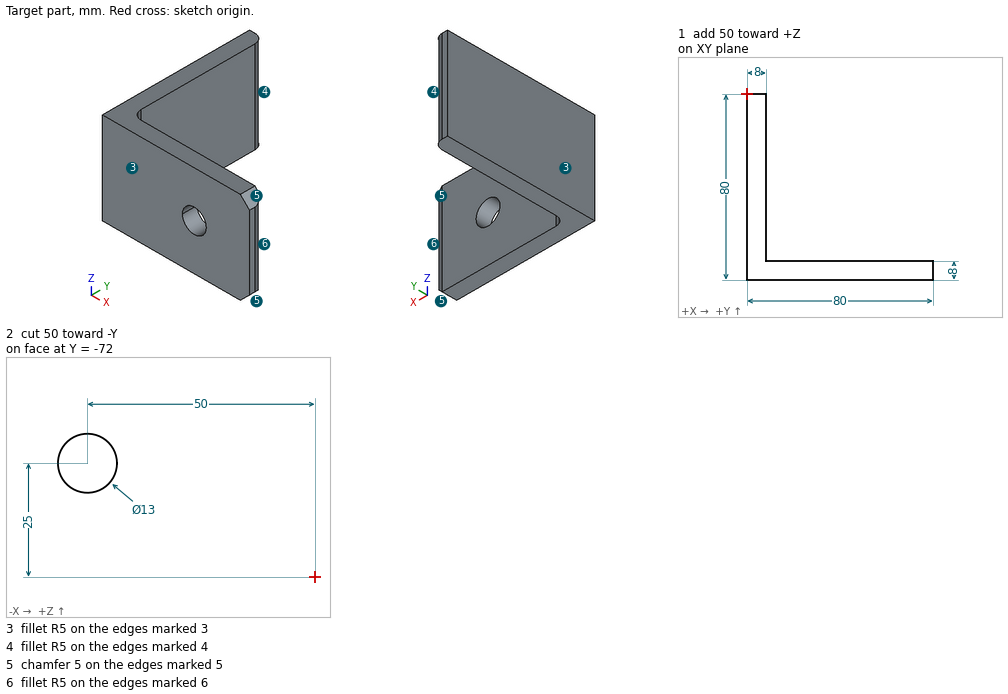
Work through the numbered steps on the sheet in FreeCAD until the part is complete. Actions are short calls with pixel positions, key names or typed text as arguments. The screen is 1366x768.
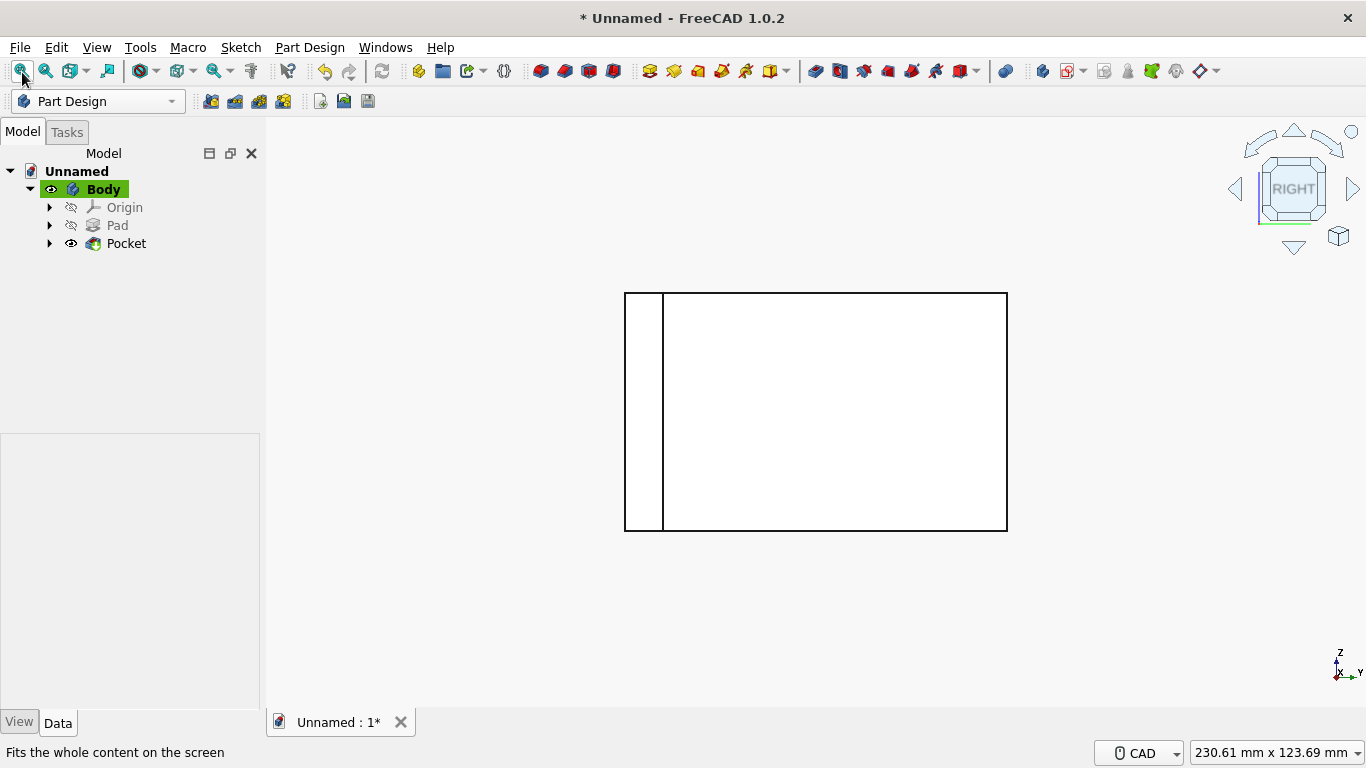
key(5)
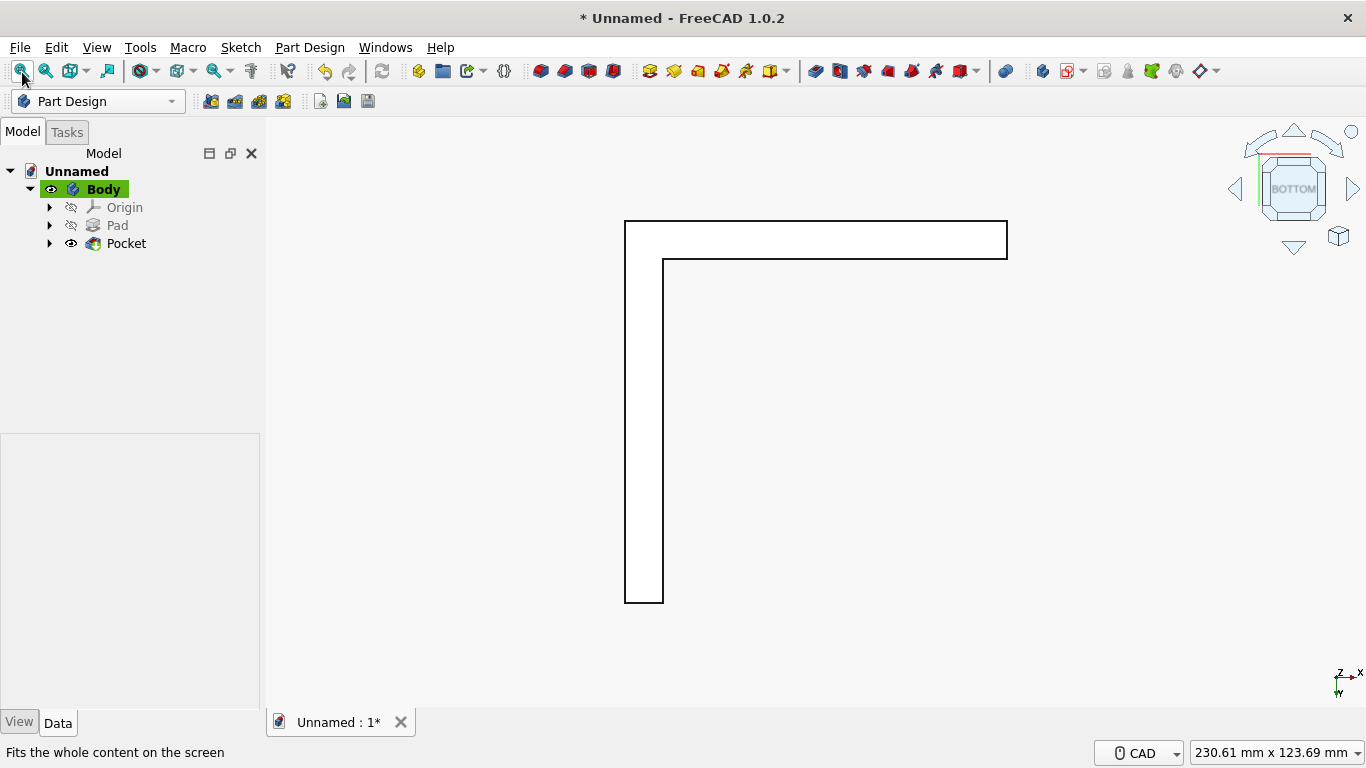
key(4)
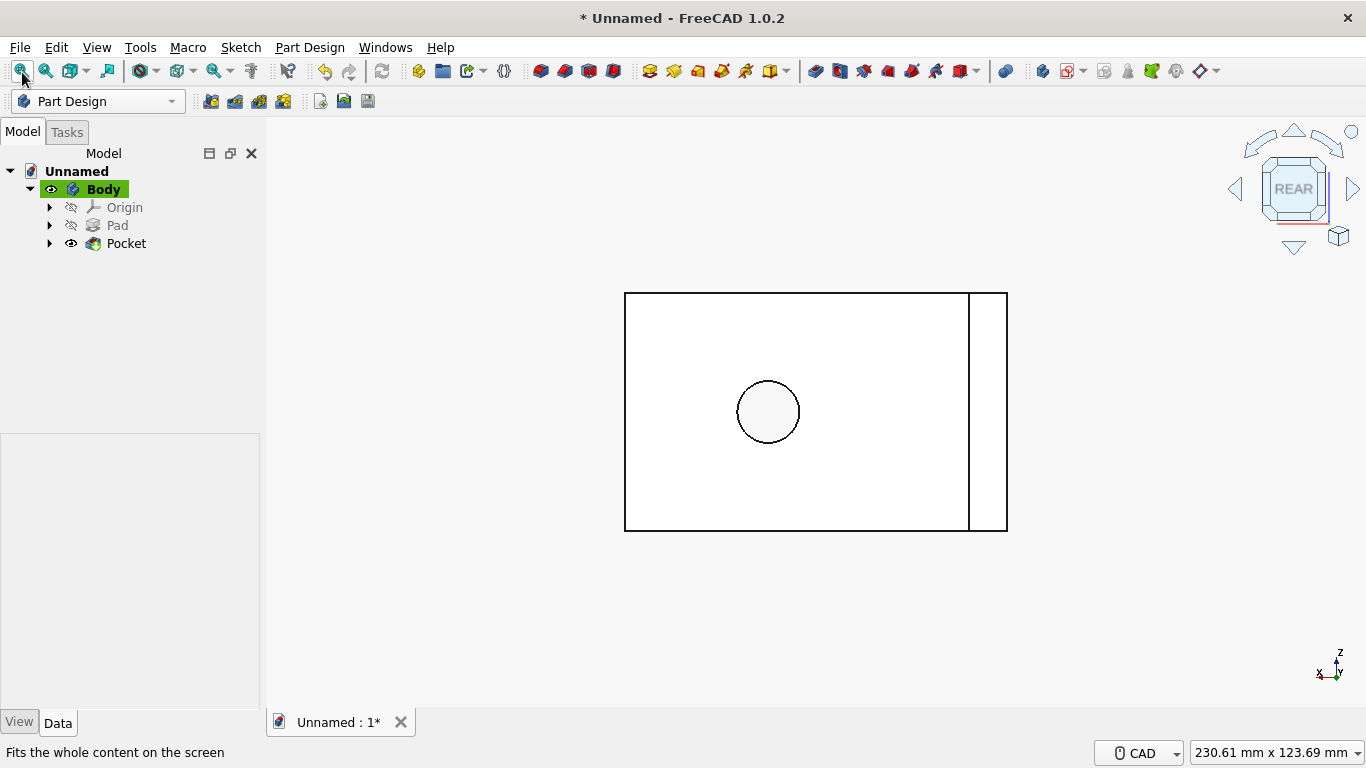
click(22, 72)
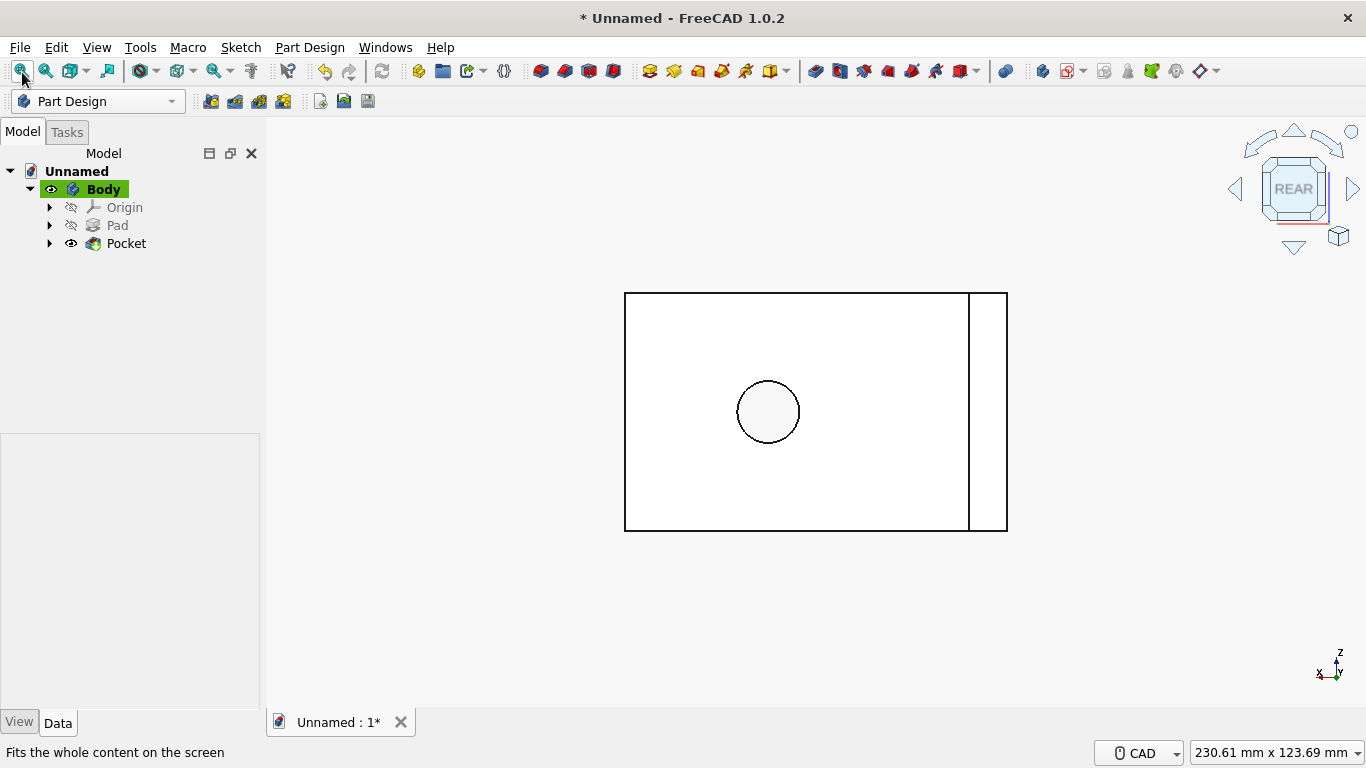
key(6)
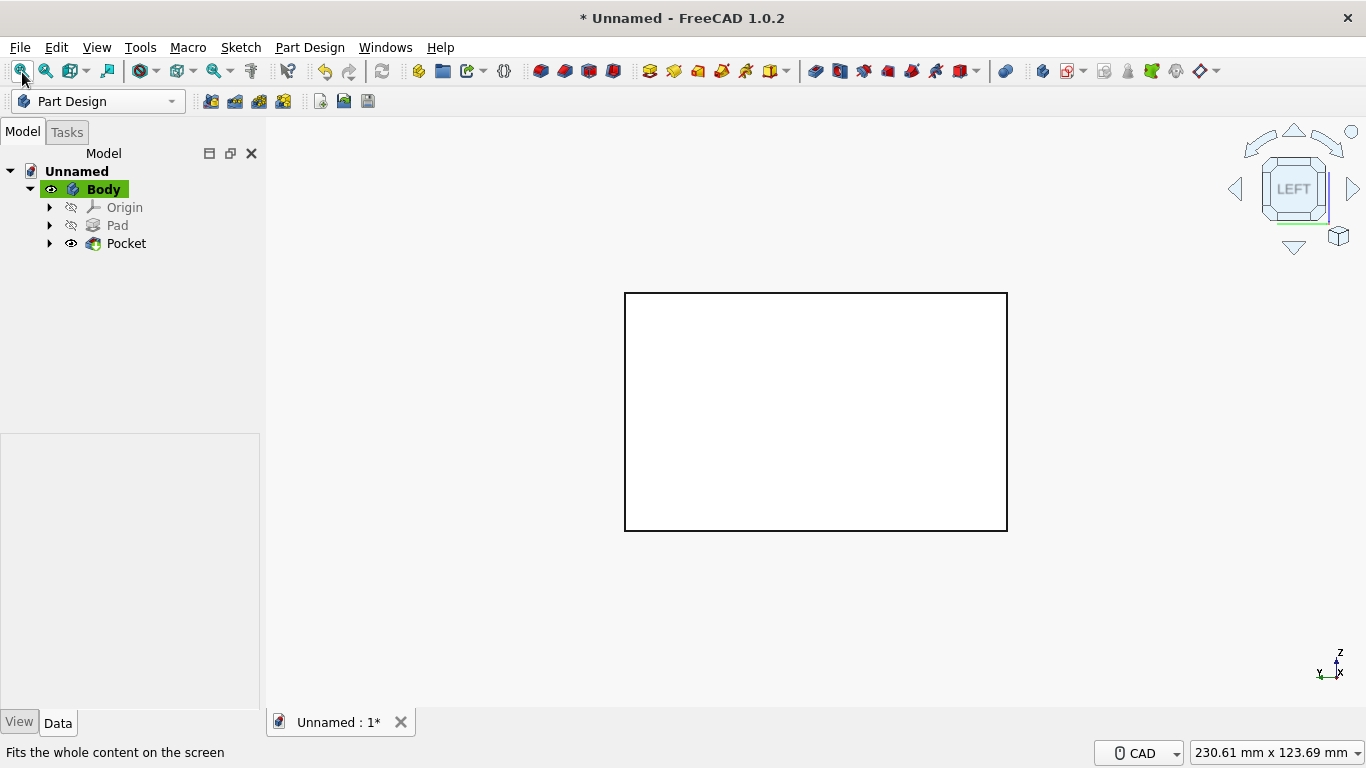
click(22, 72)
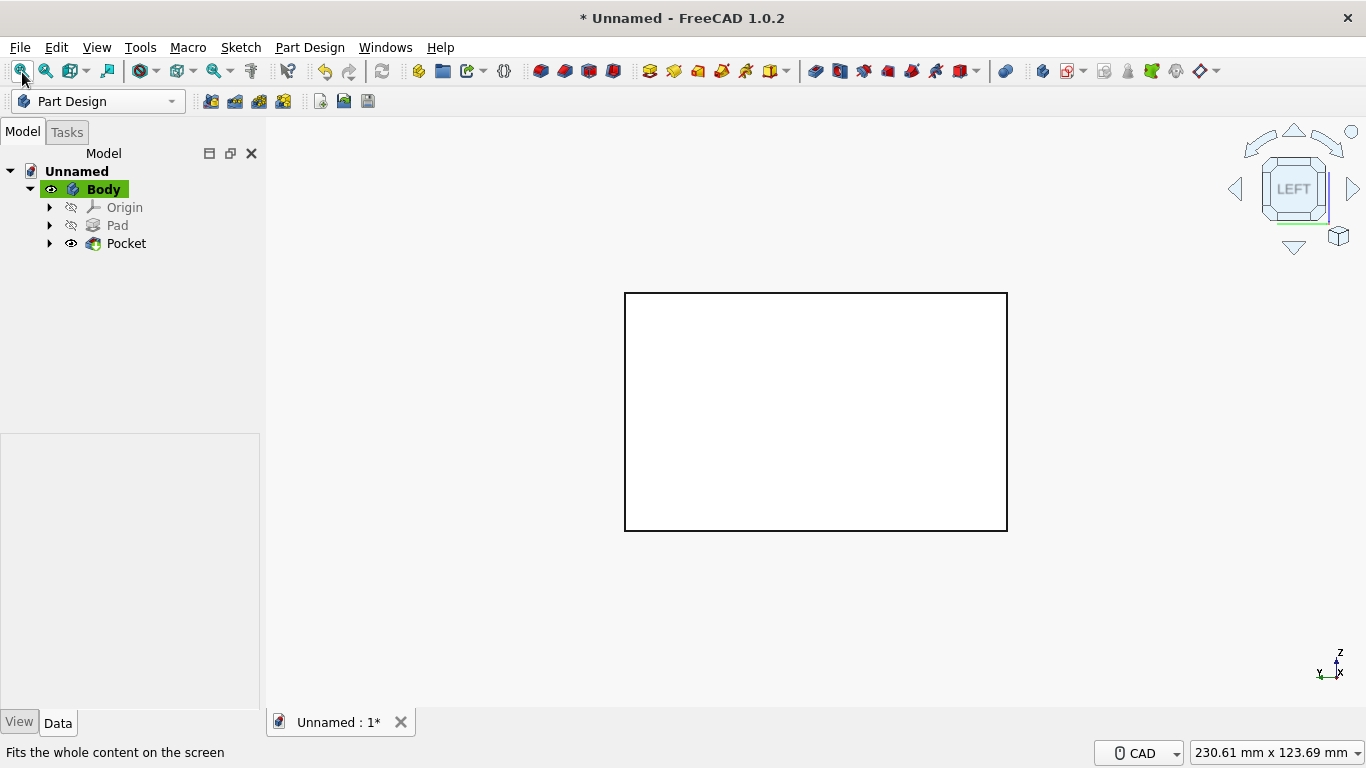
key(v)
key(3)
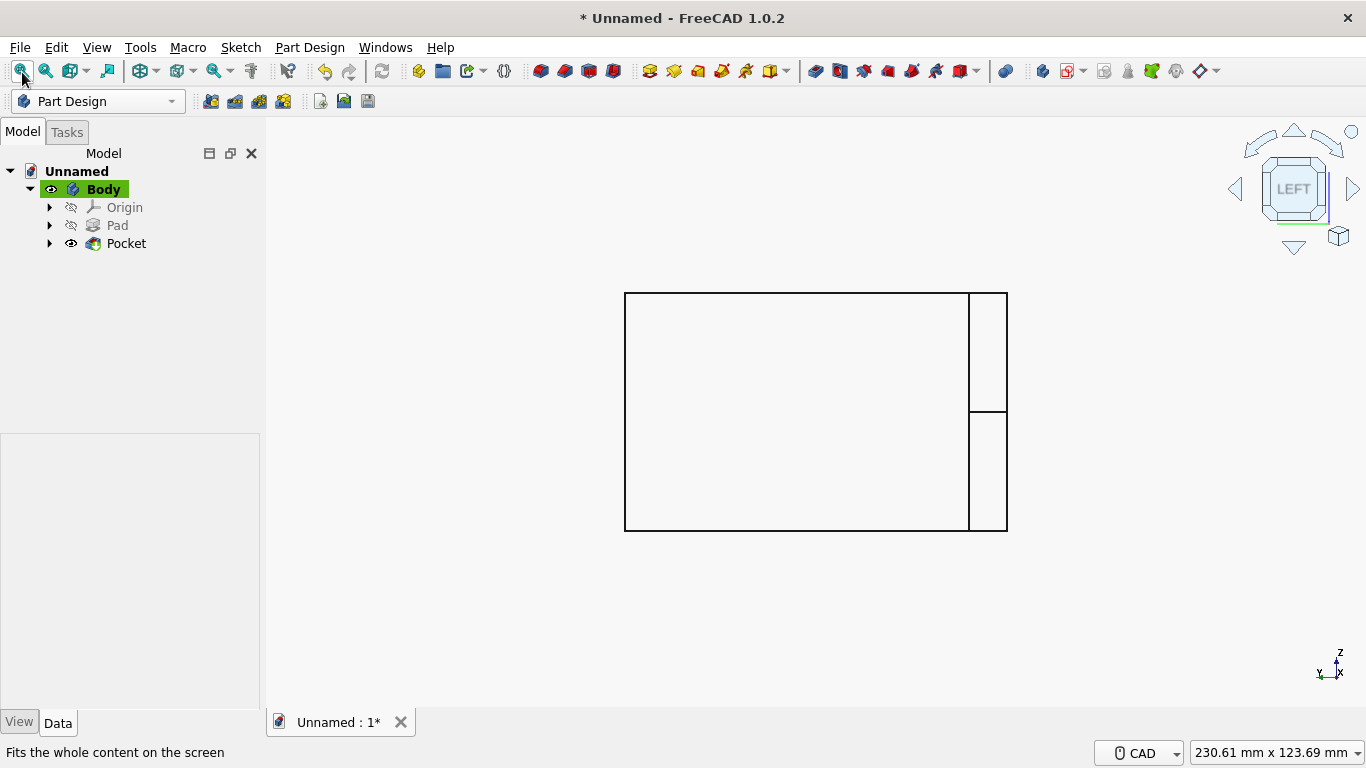
key(0)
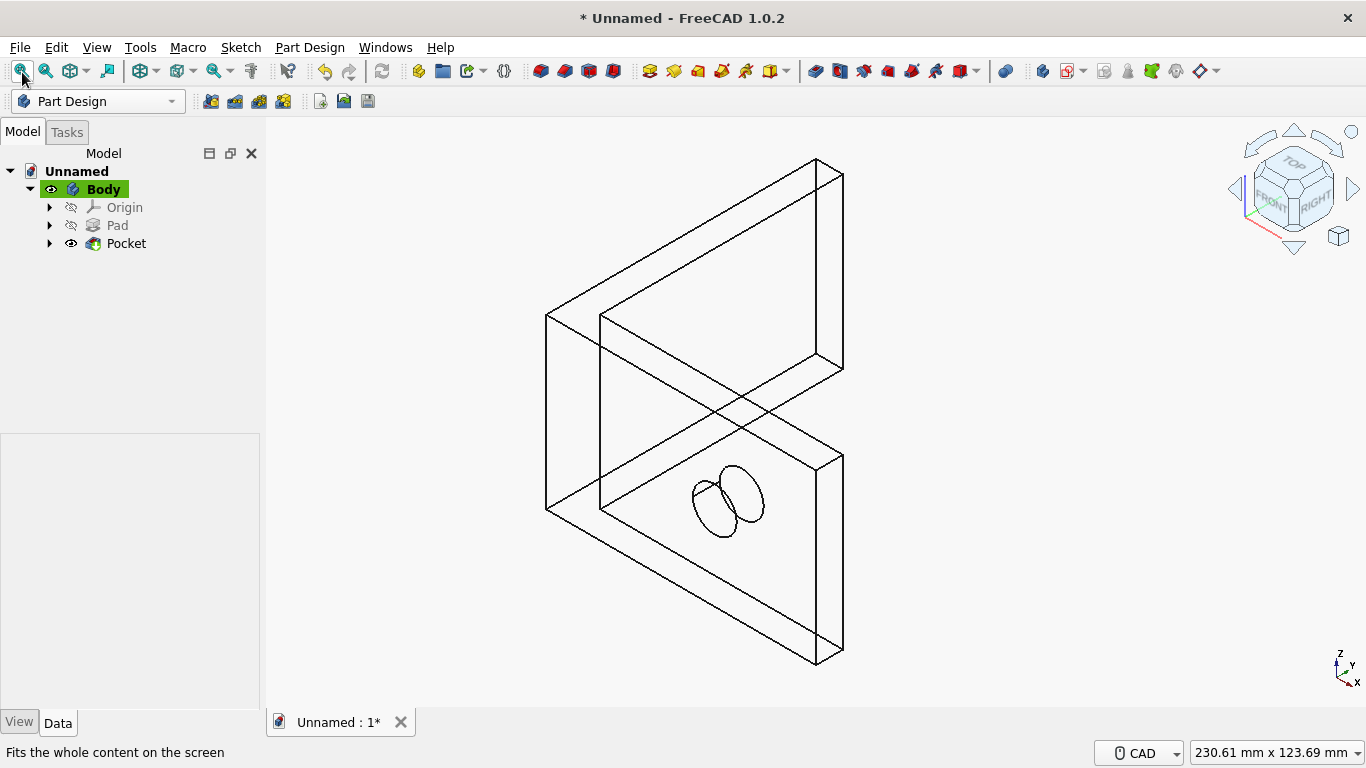
click(600, 411)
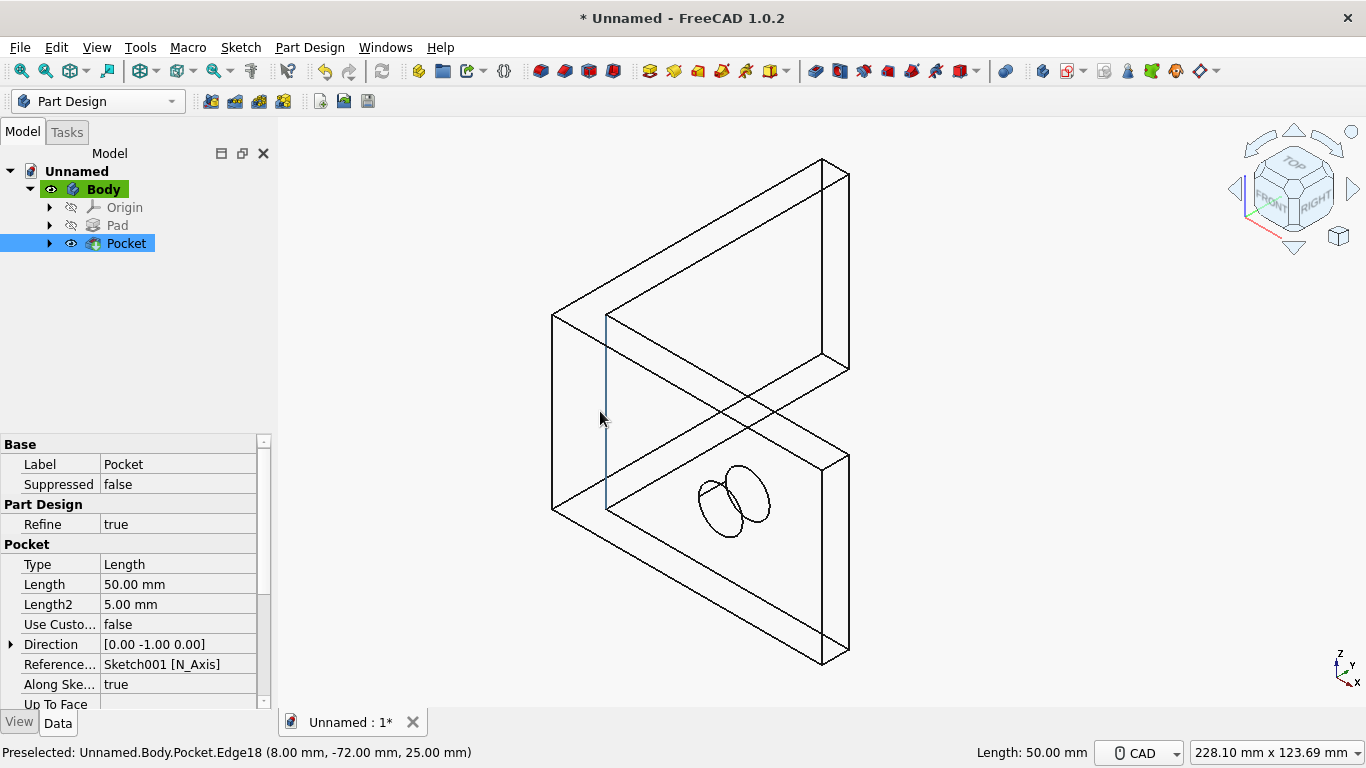
key(v)
key(1)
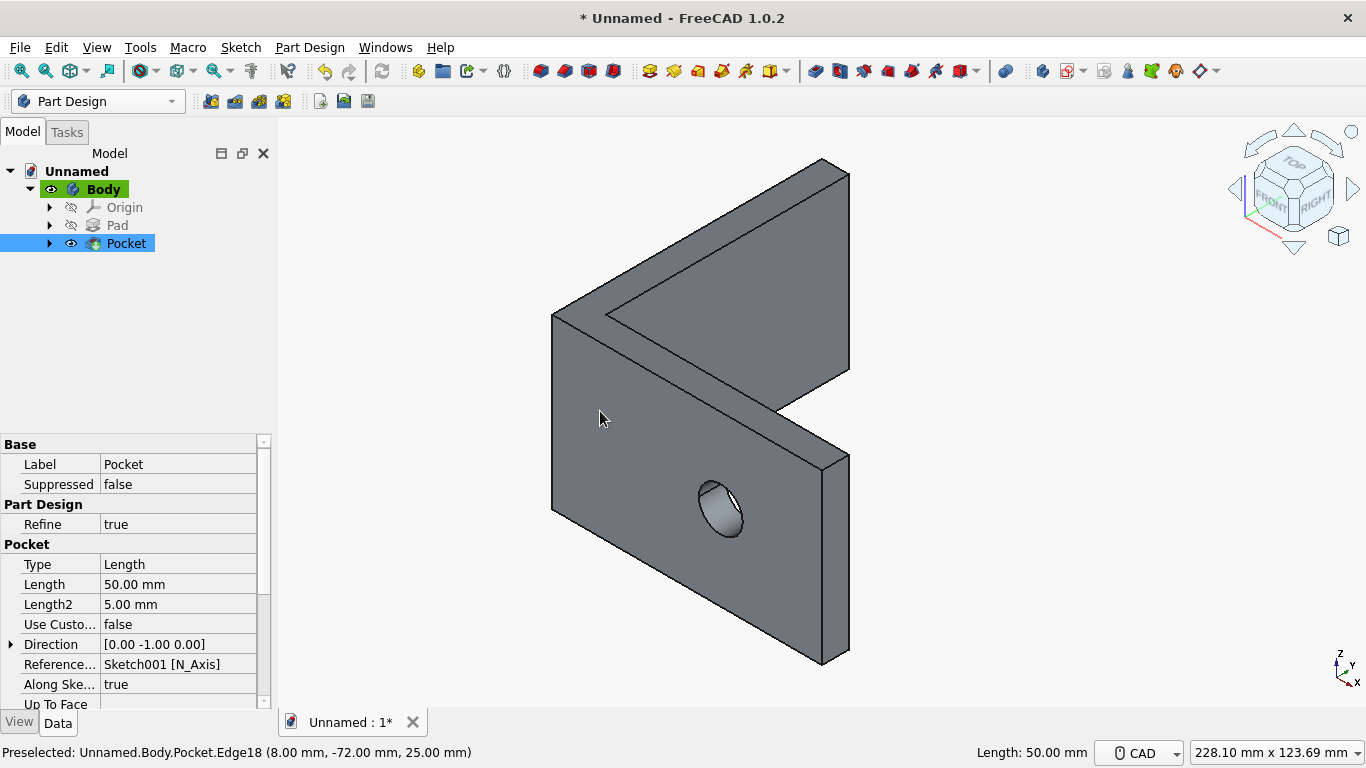
click(542, 72)